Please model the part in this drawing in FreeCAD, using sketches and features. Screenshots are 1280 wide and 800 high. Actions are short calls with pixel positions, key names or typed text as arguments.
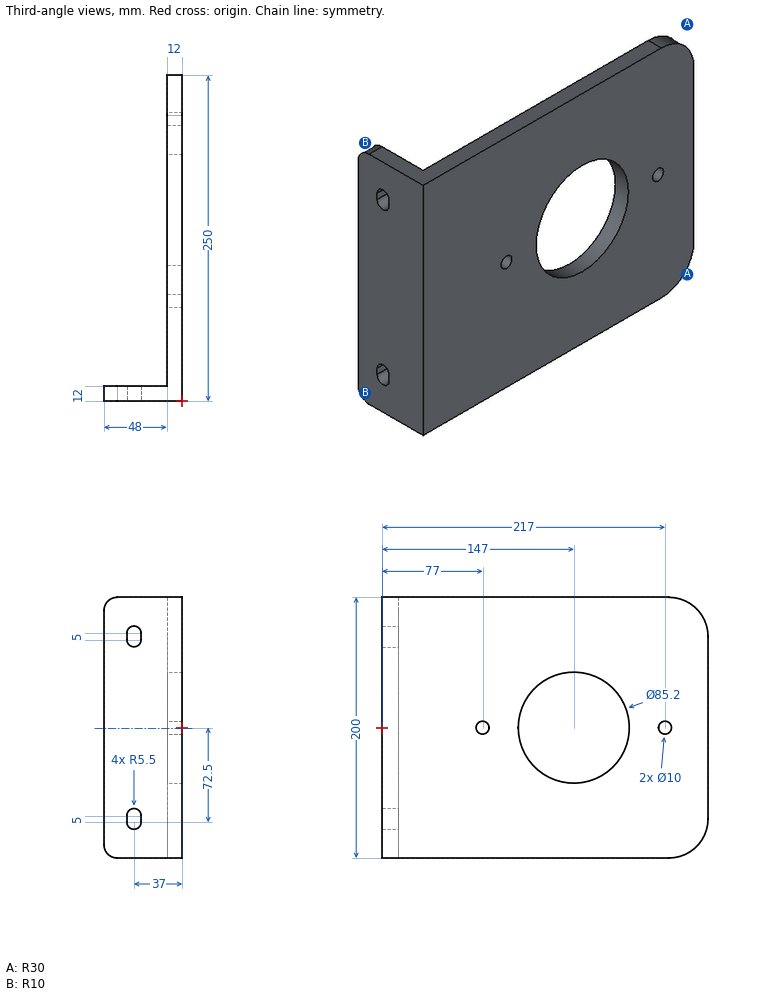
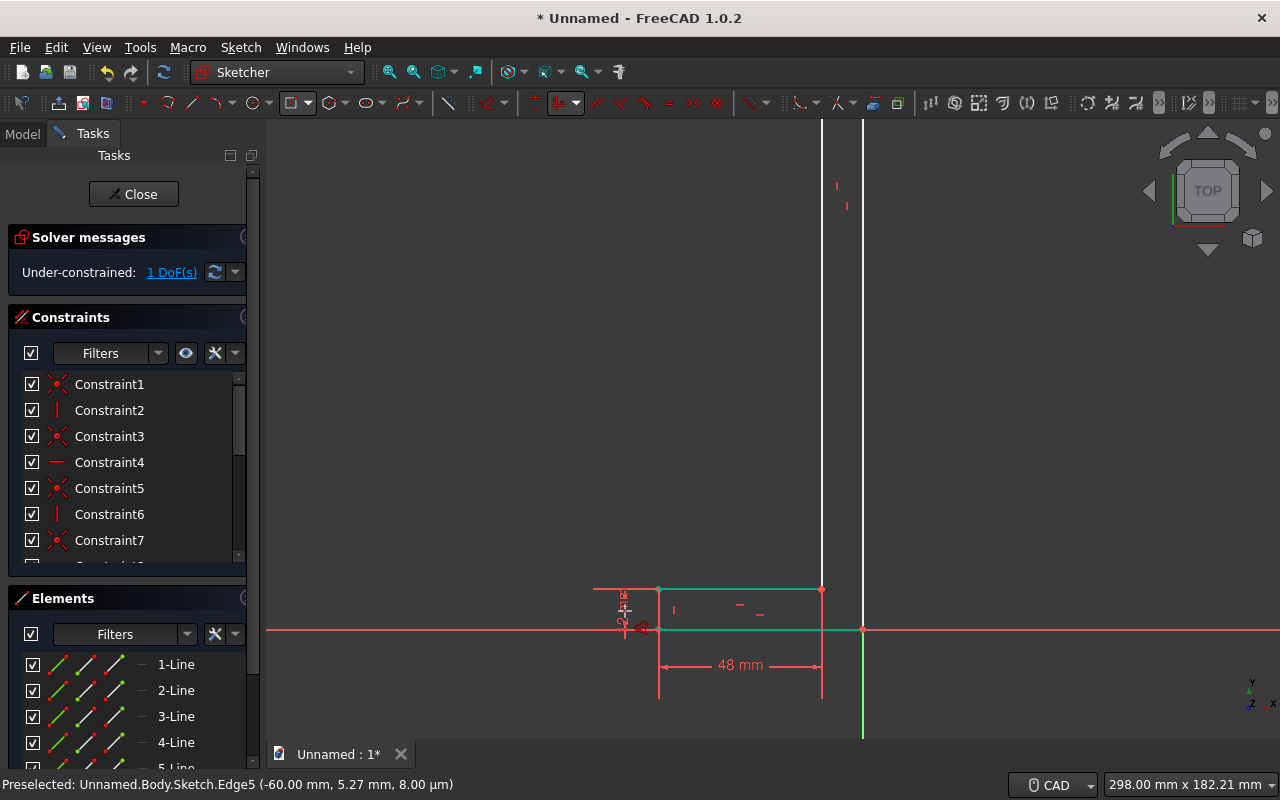
click(863, 376)
click(897, 388)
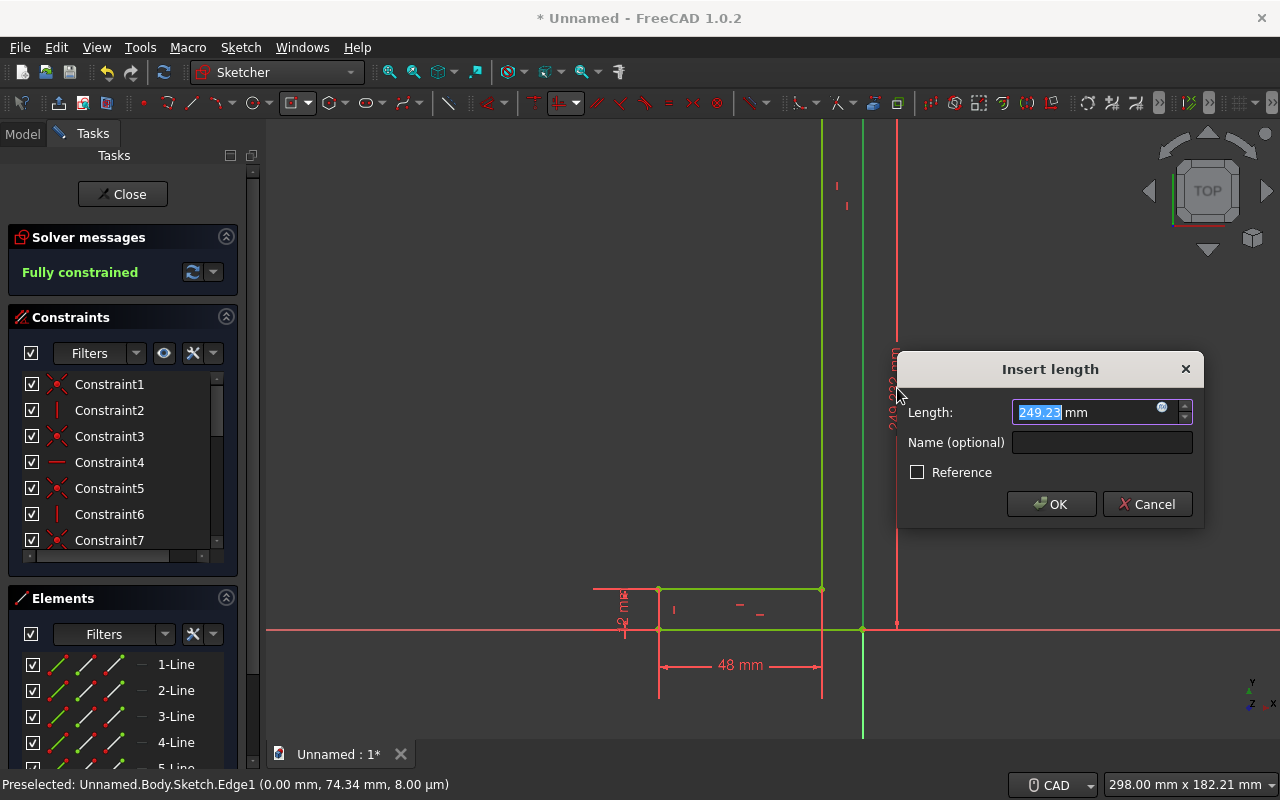
text(250)
key(Return)
key(Escape)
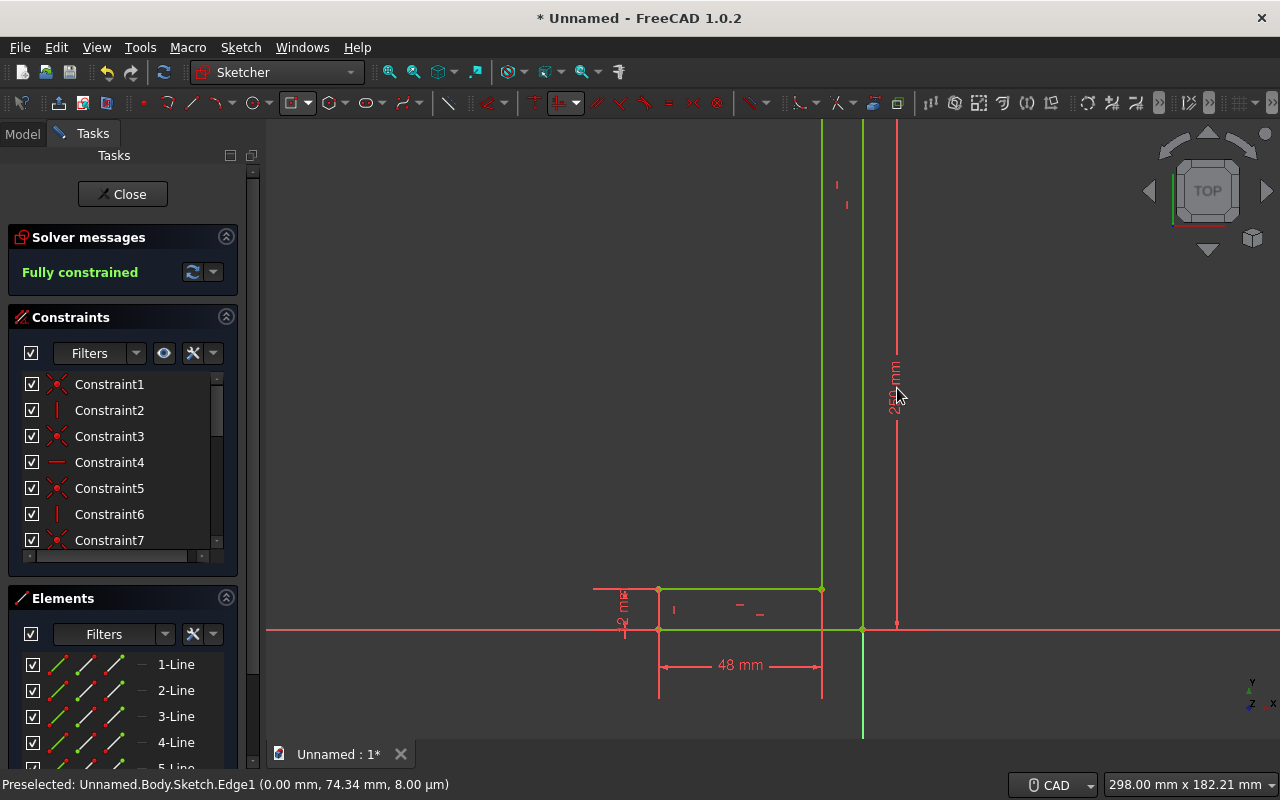
click(123, 194)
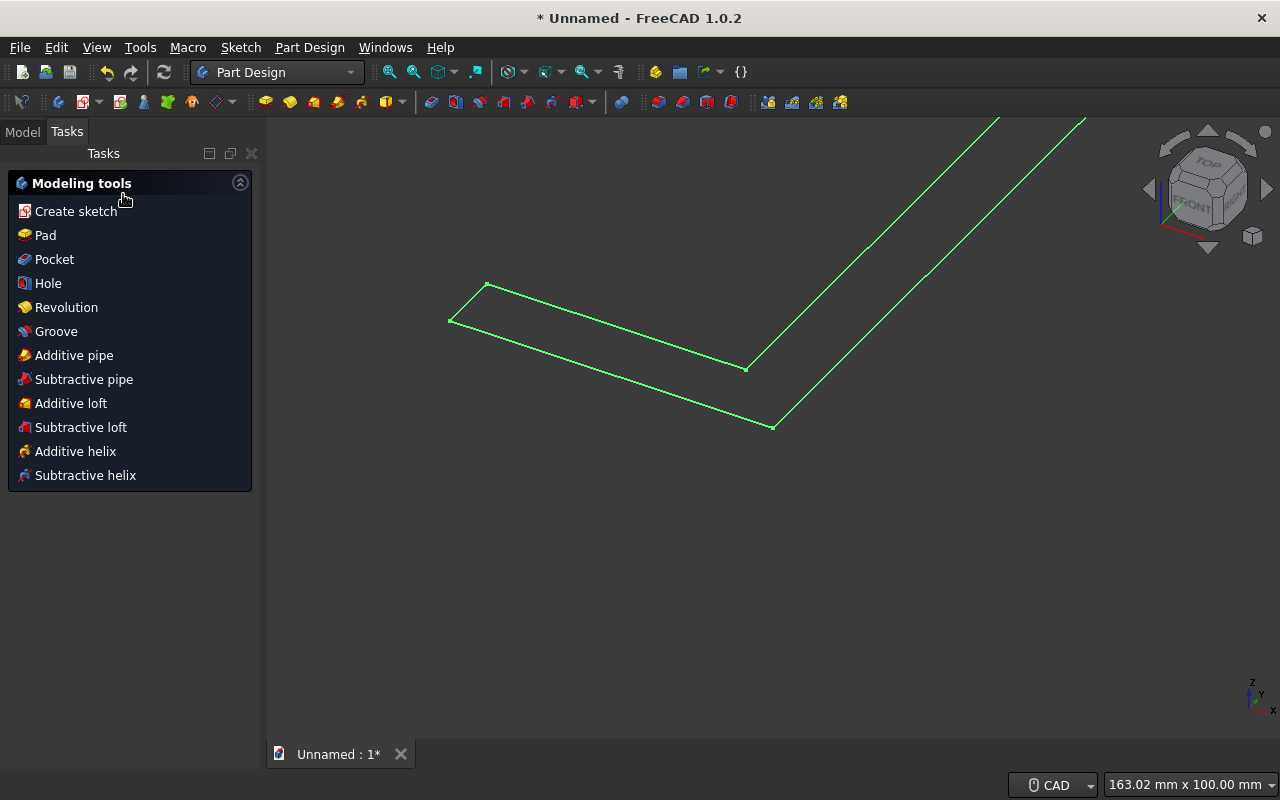
click(266, 102)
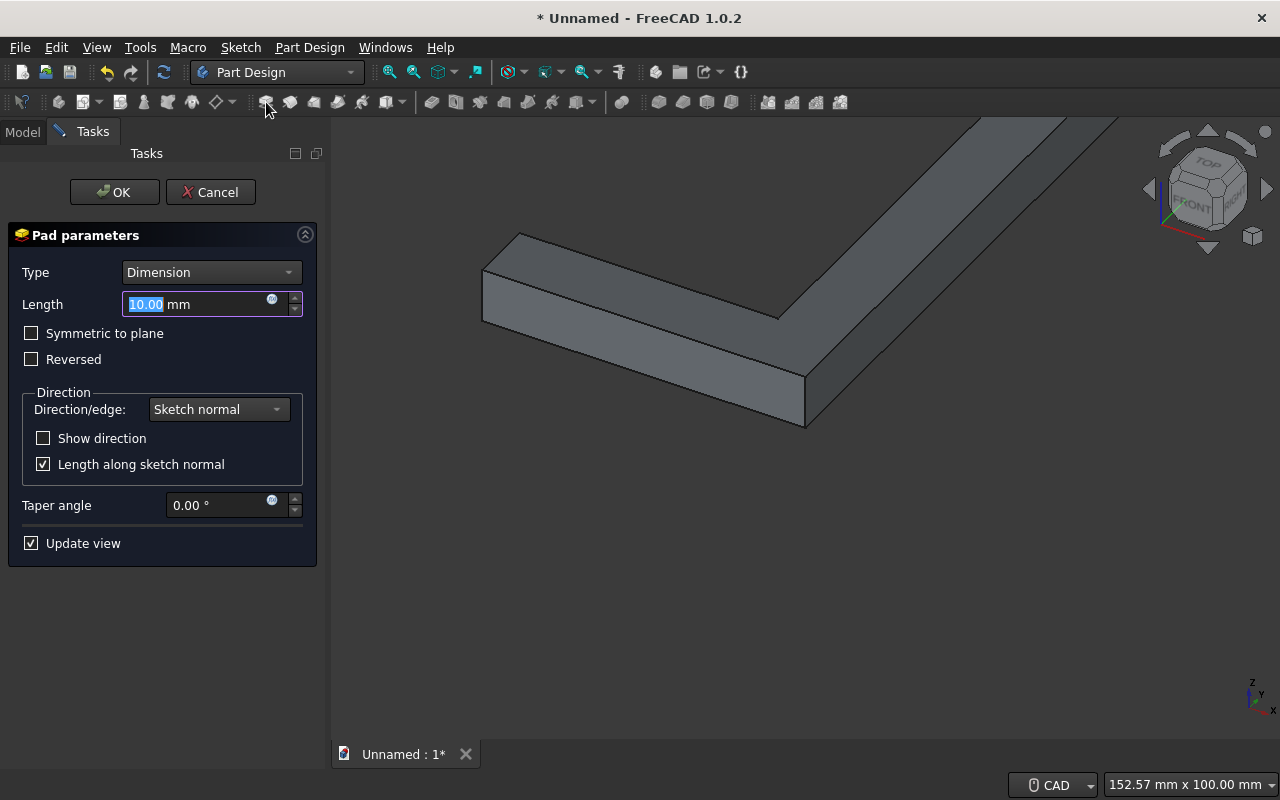
text(200)
key(Tab)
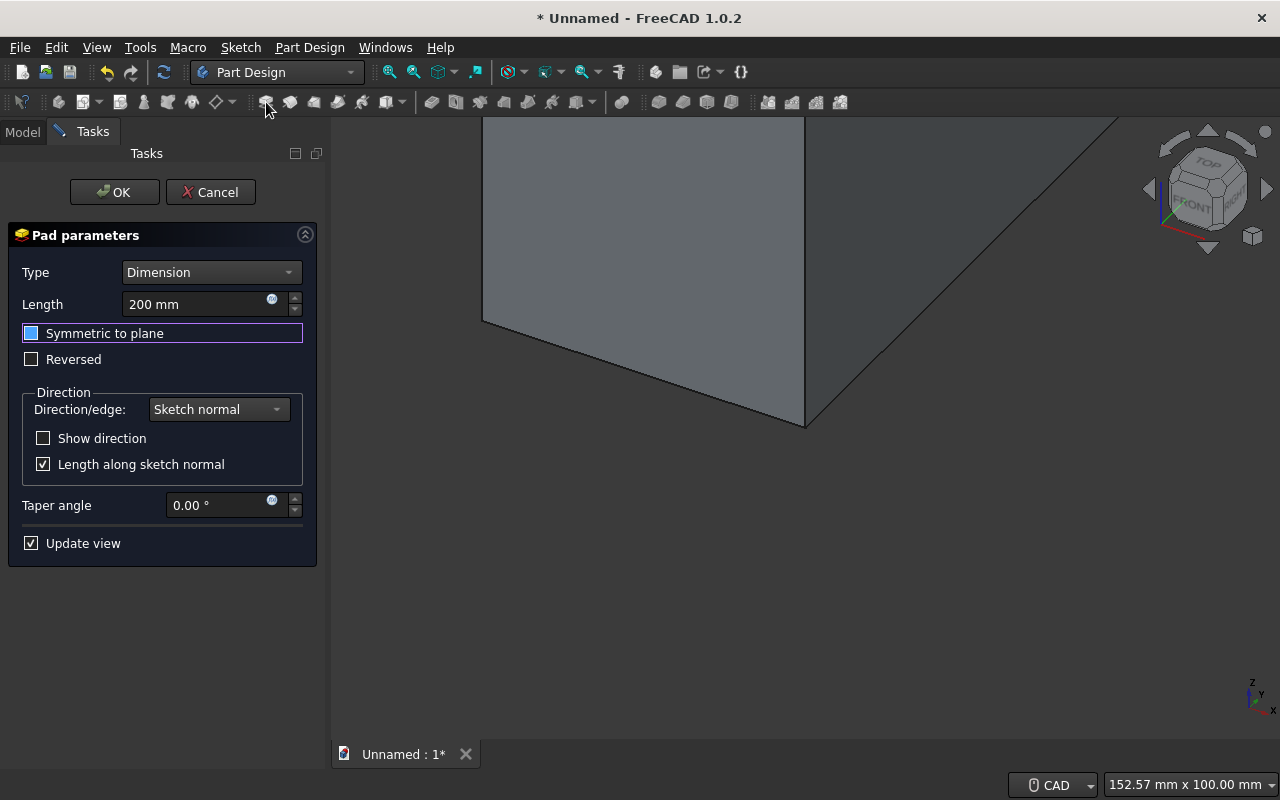
click(30, 333)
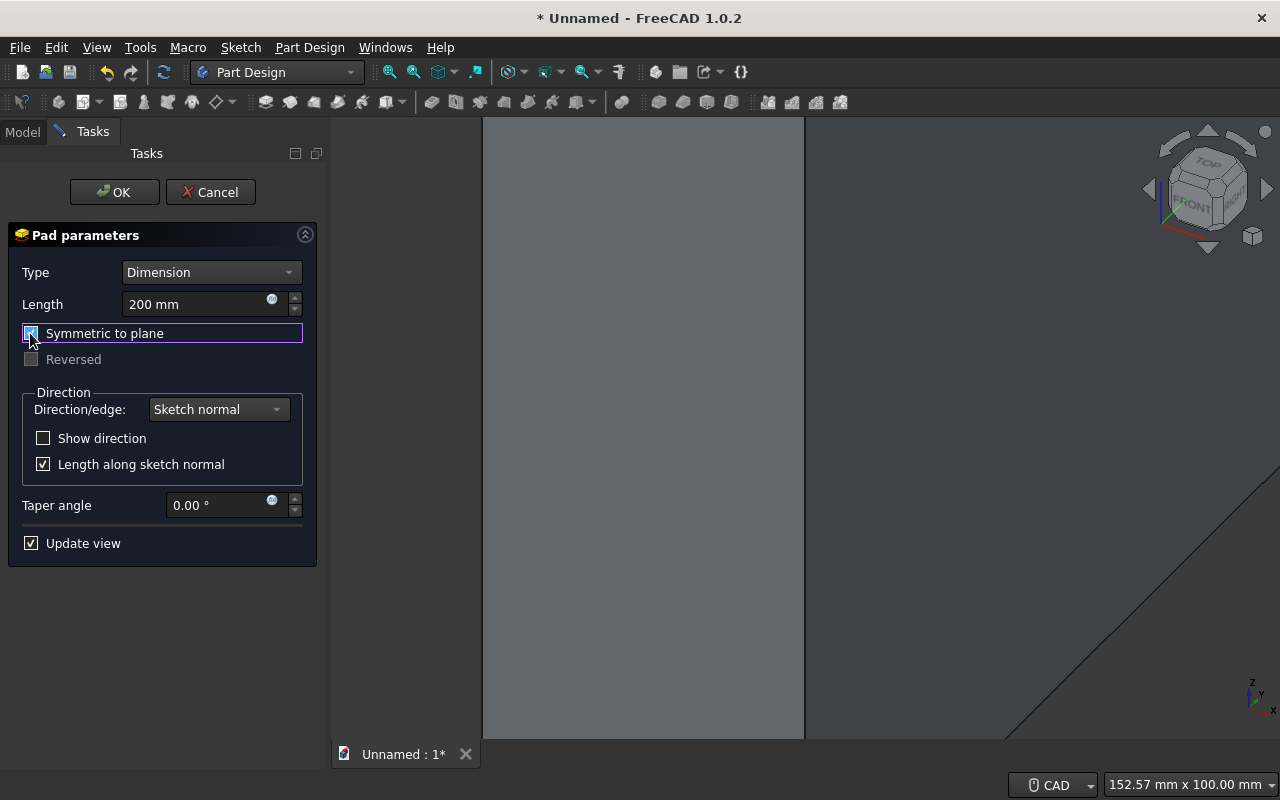
click(115, 192)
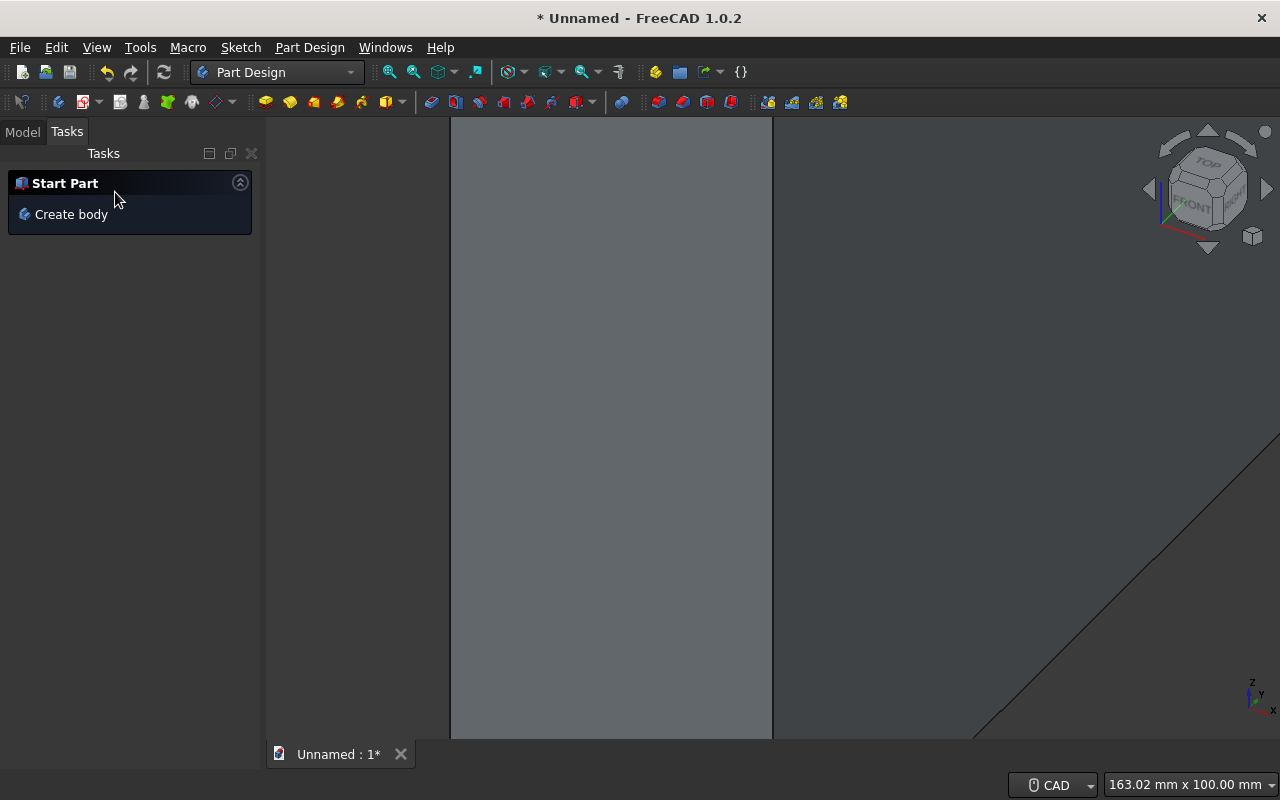
click(390, 72)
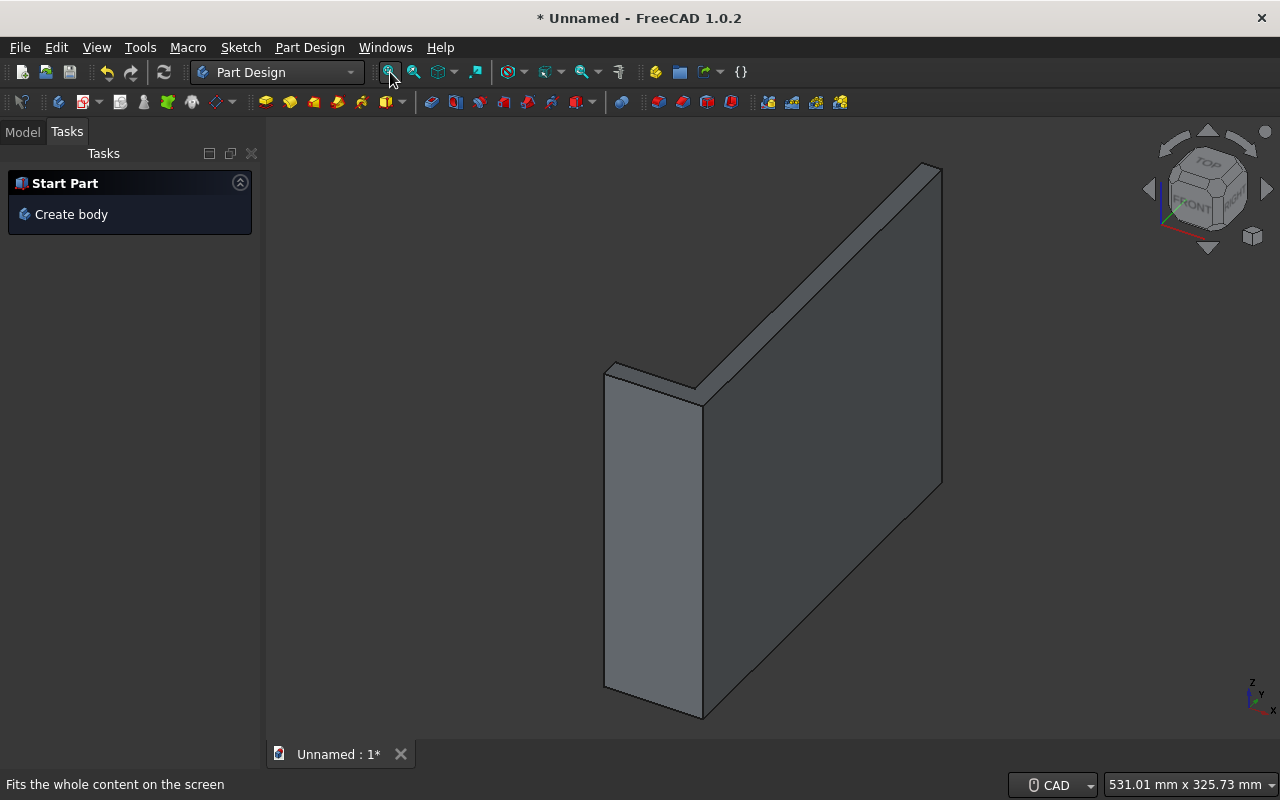
key(4)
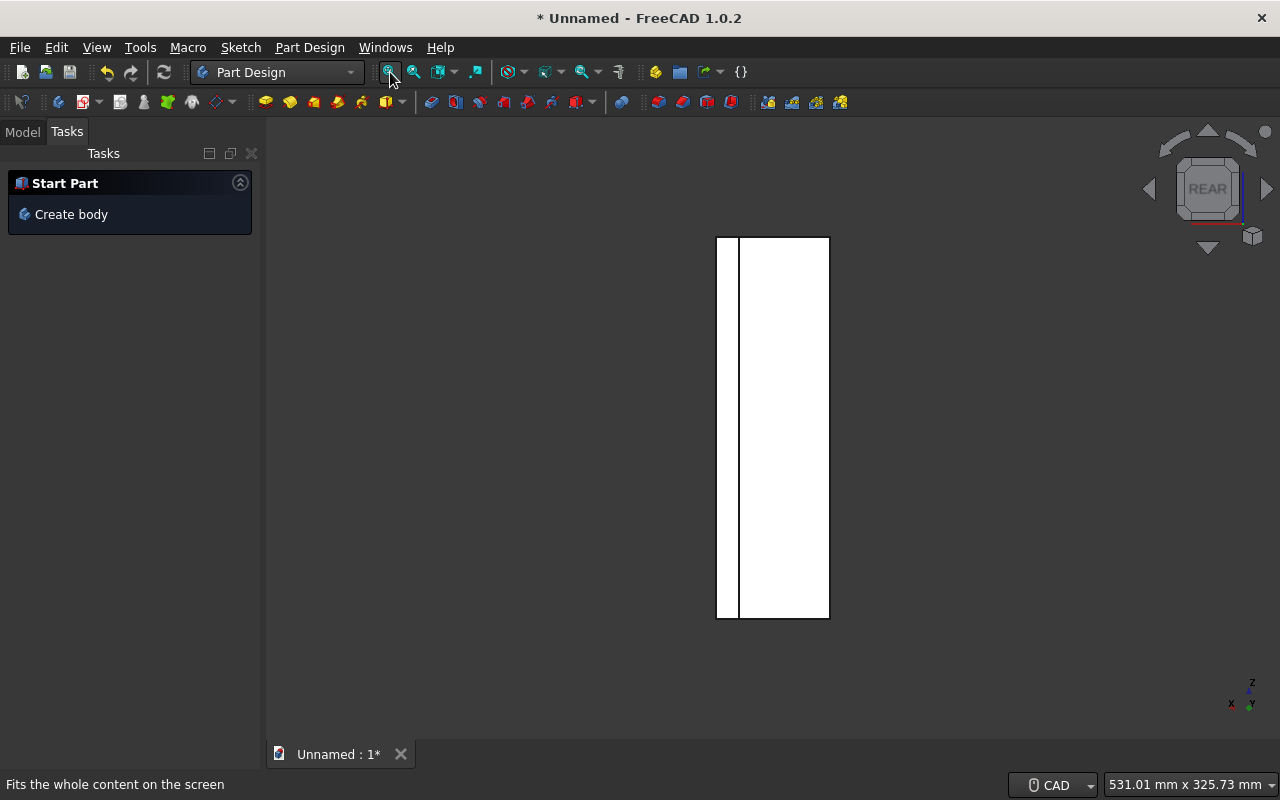
click(784, 318)